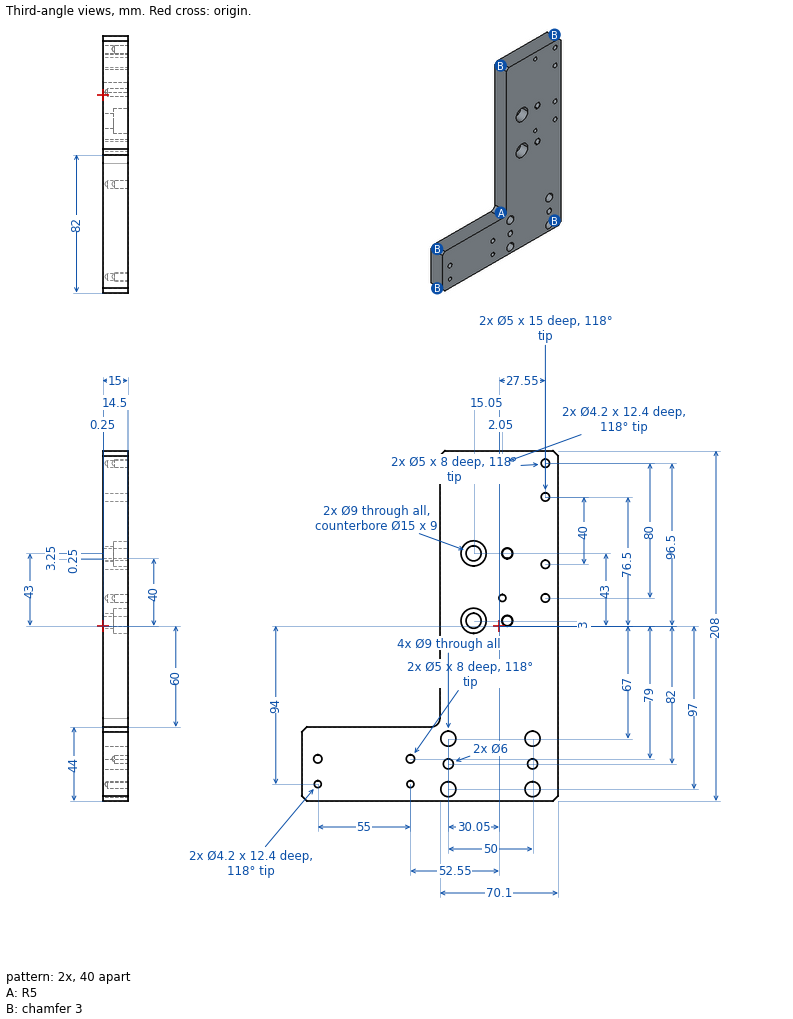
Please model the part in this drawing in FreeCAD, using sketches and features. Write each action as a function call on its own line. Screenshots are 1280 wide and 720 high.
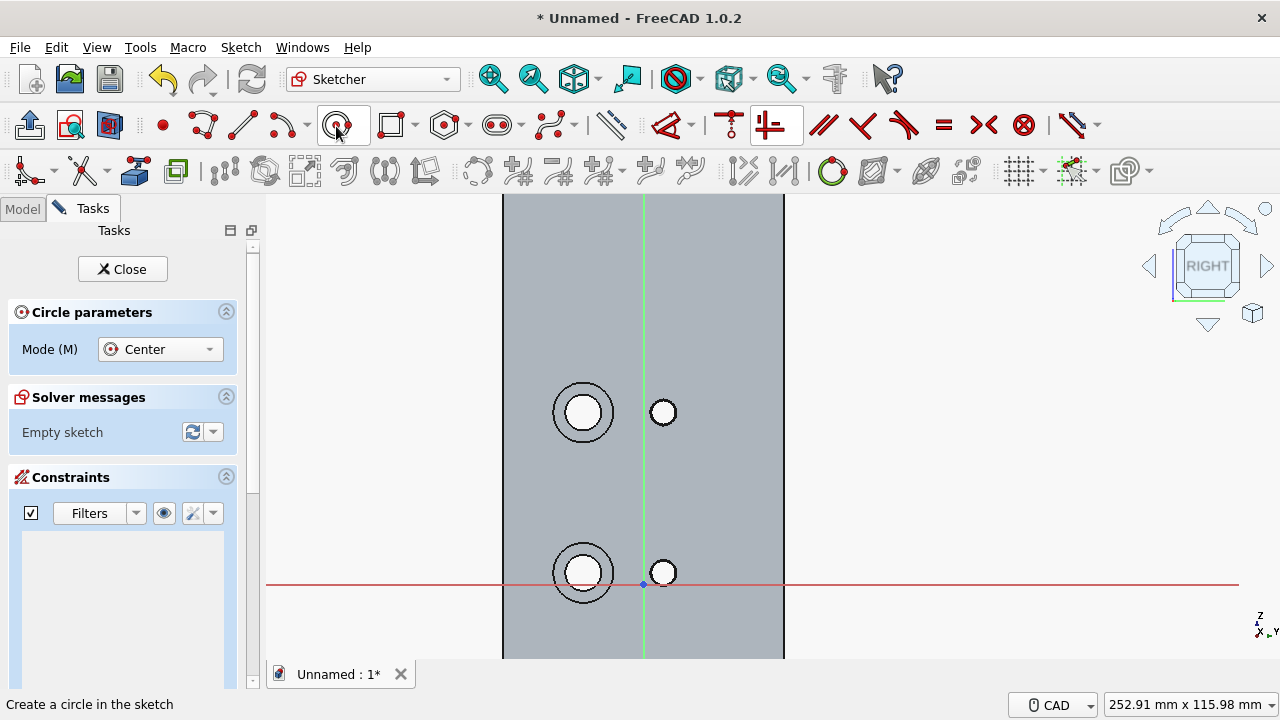
scroll(754, 278, up, 5)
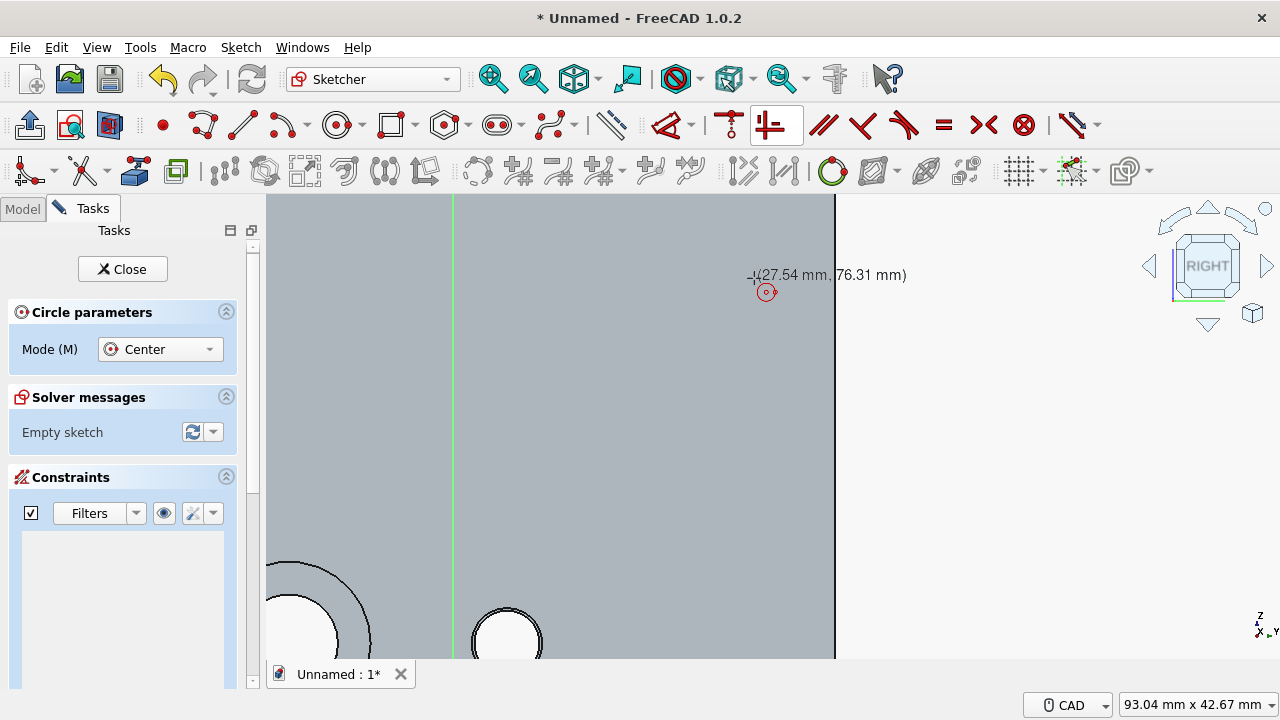
click(753, 278)
click(773, 259)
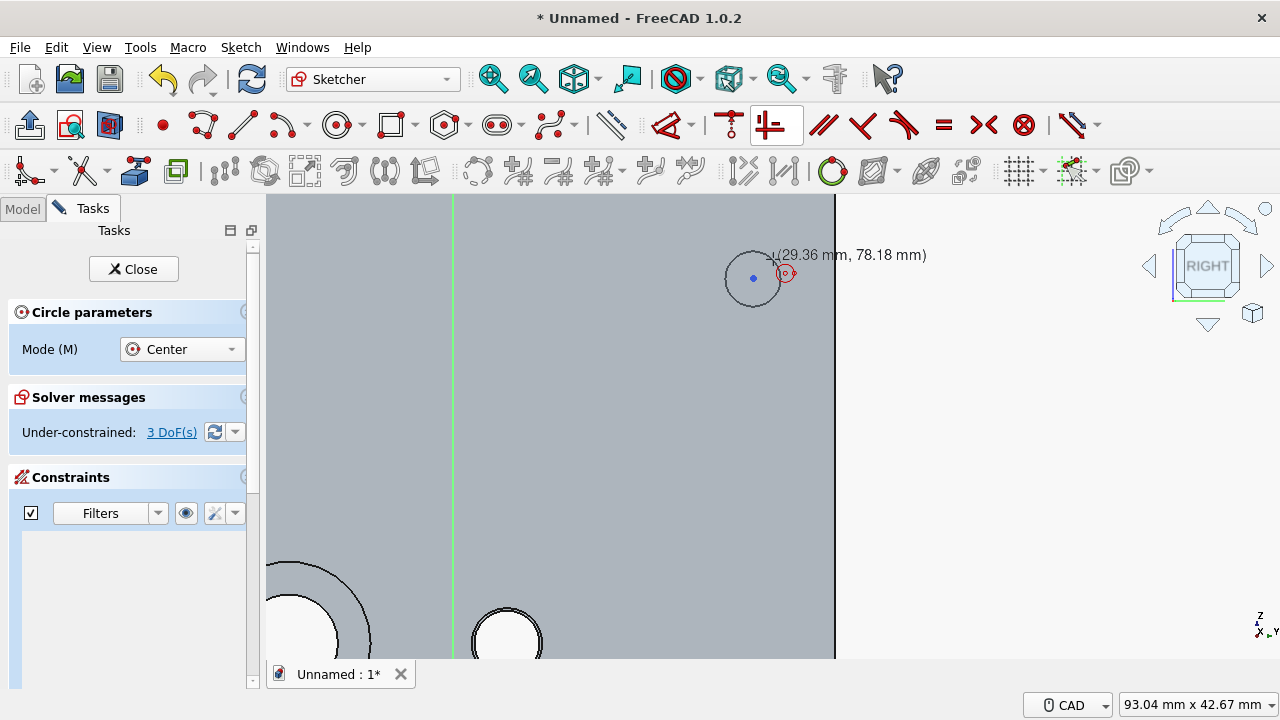
scroll(756, 278, down, 5)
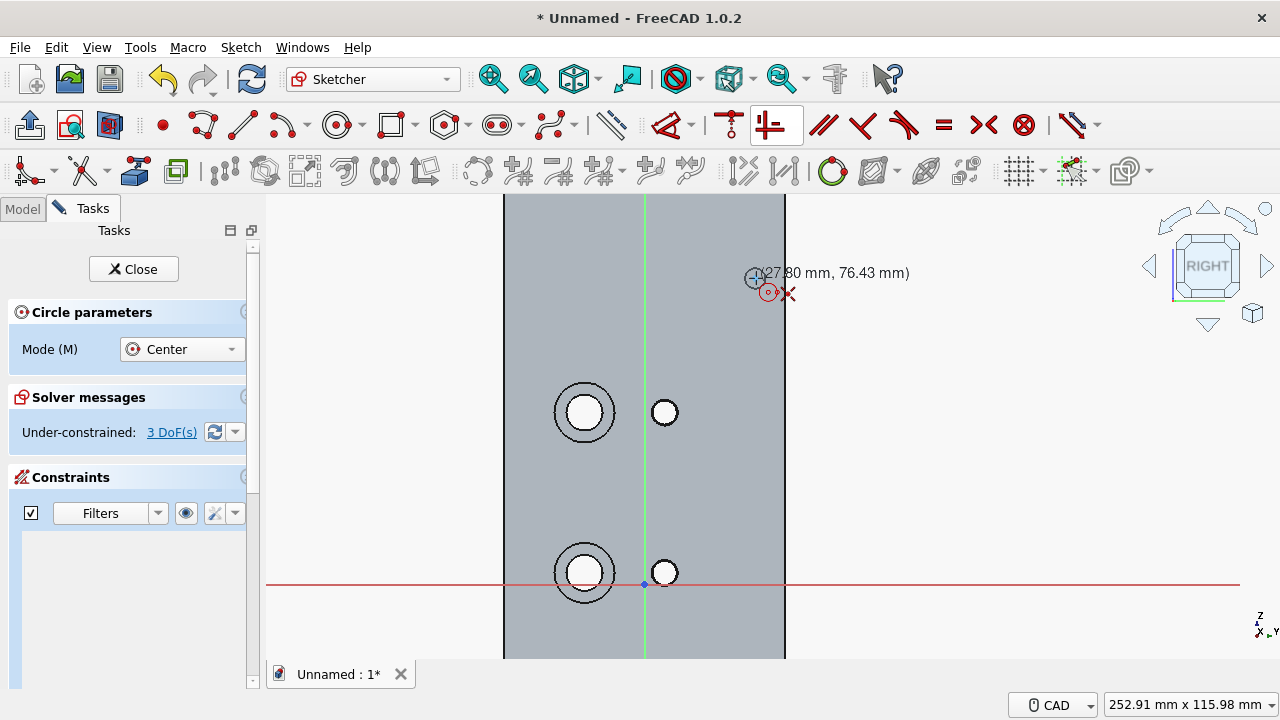
scroll(755, 439, up, 5)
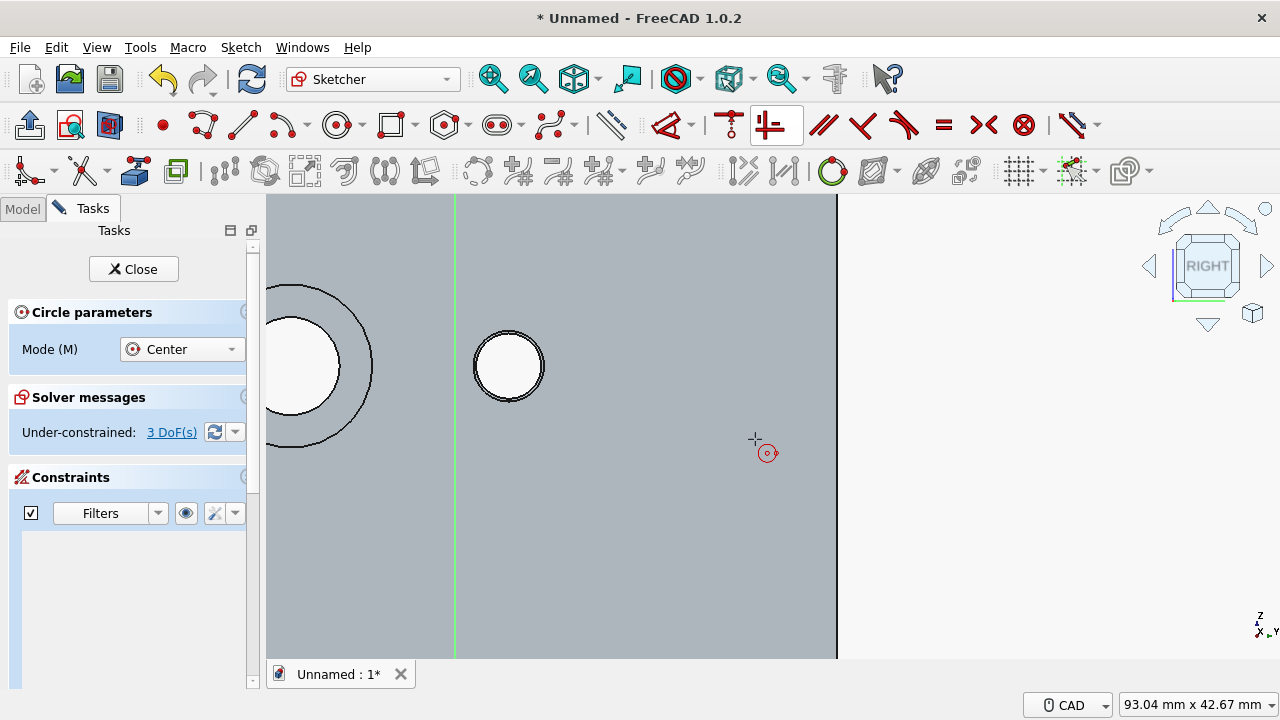
click(755, 437)
click(774, 418)
key(Escape)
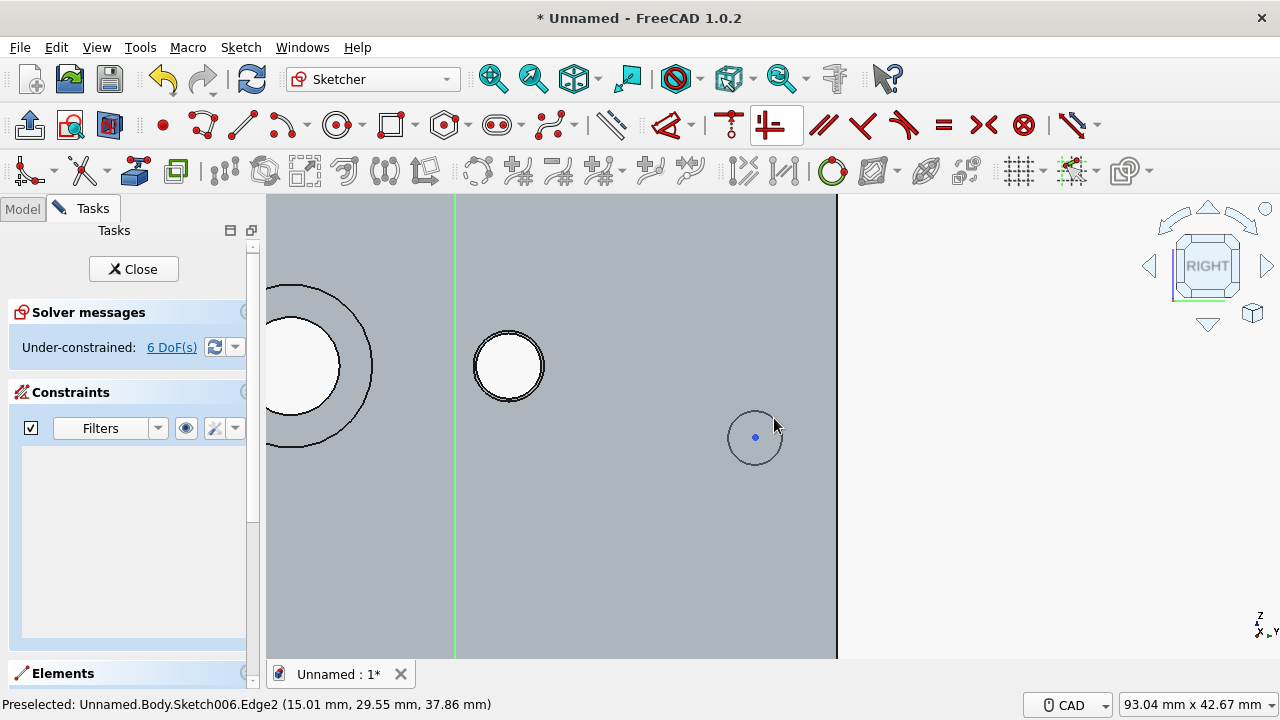
scroll(755, 439, down, 5)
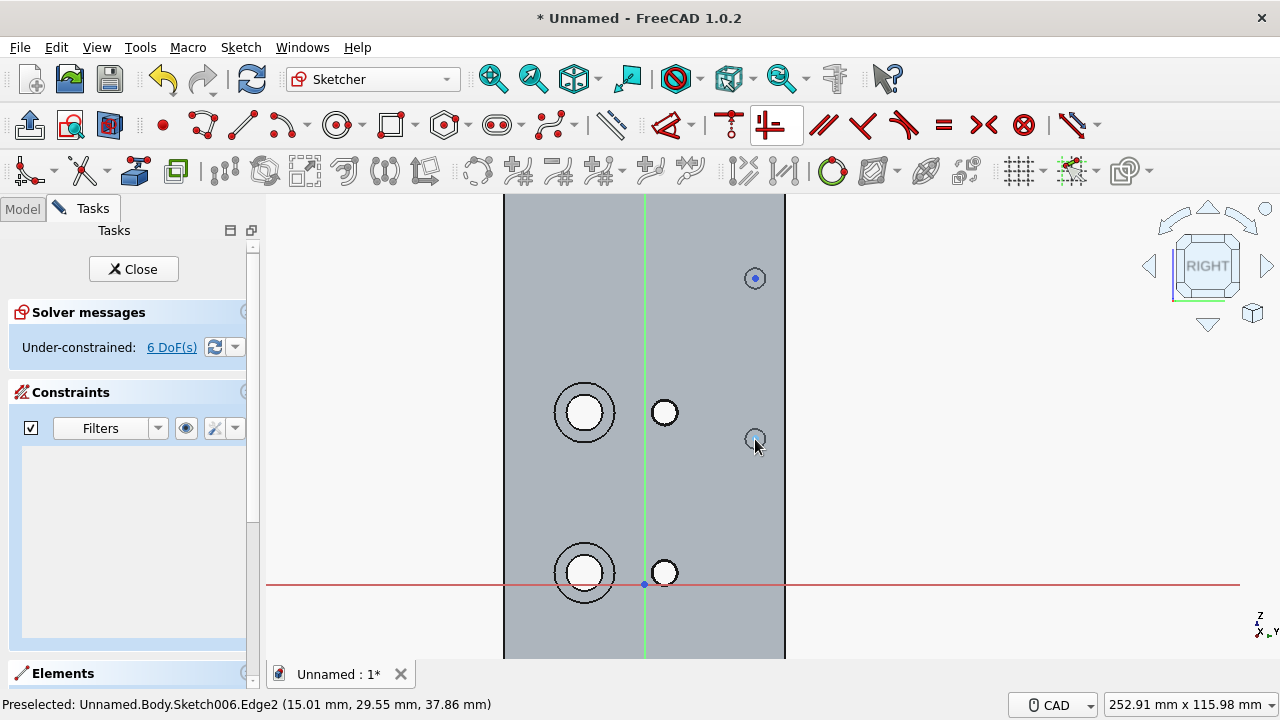
scroll(762, 271, up, 2)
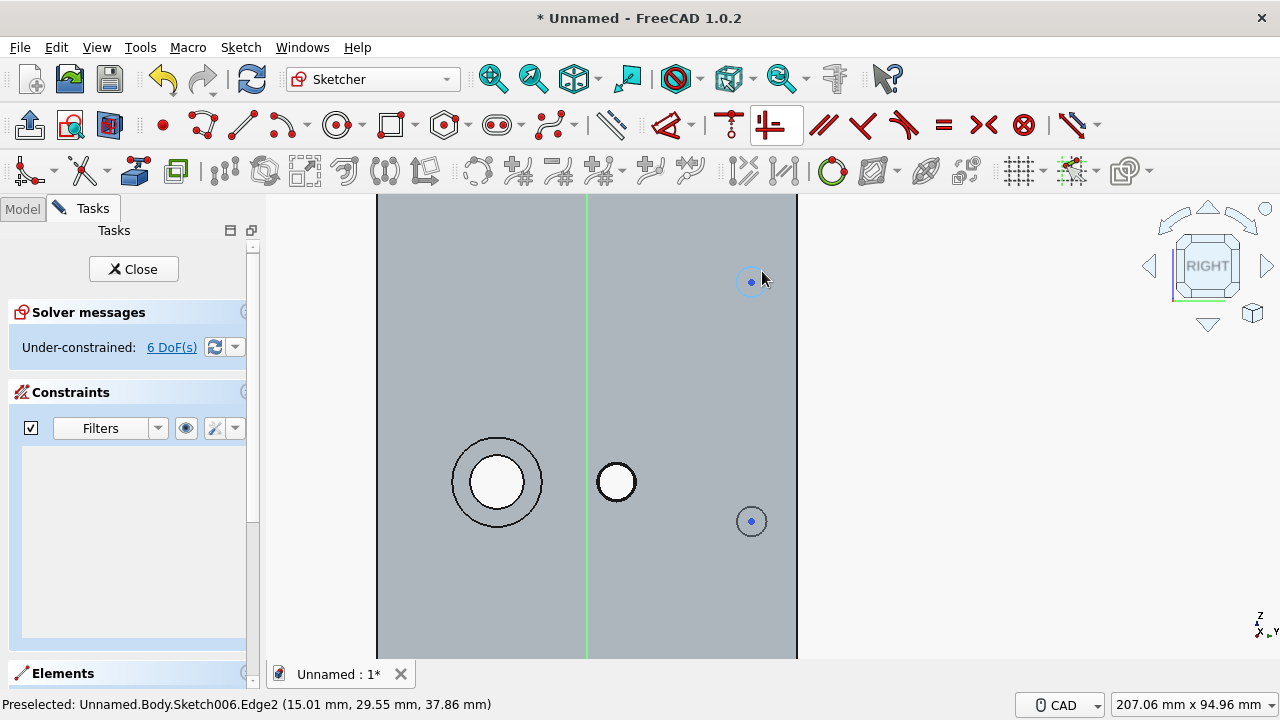
click(762, 271)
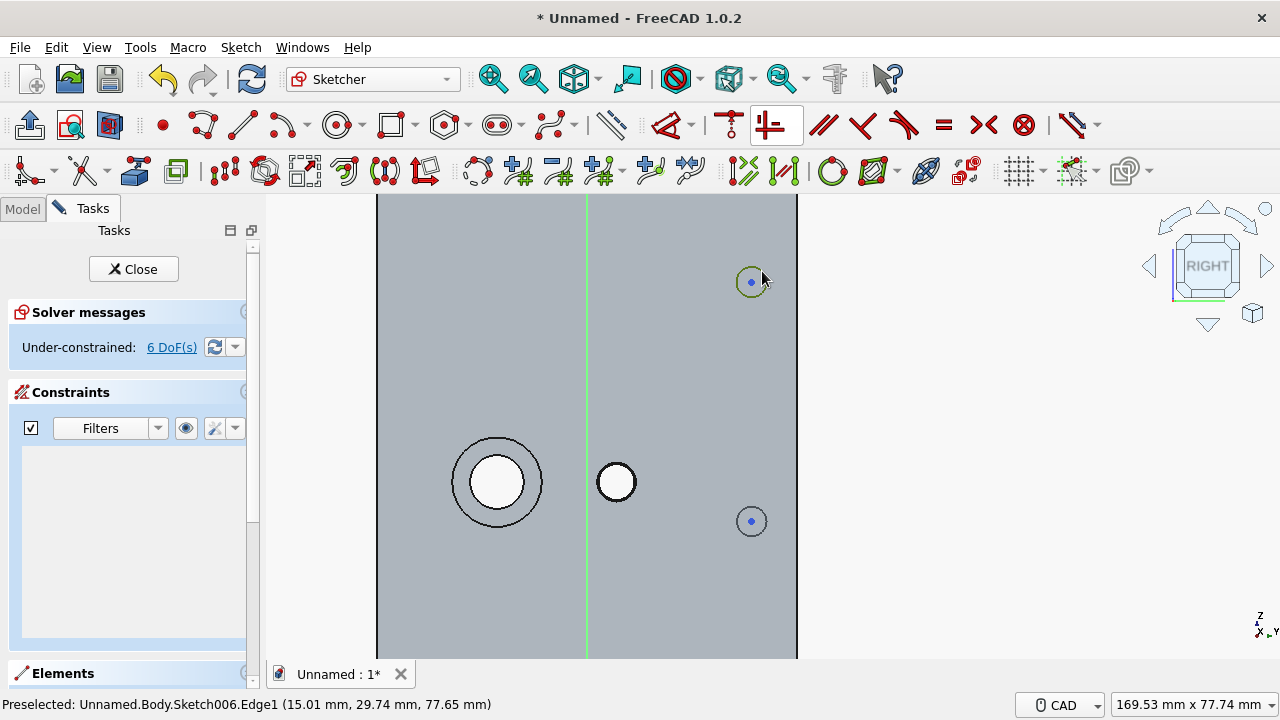
click(762, 511)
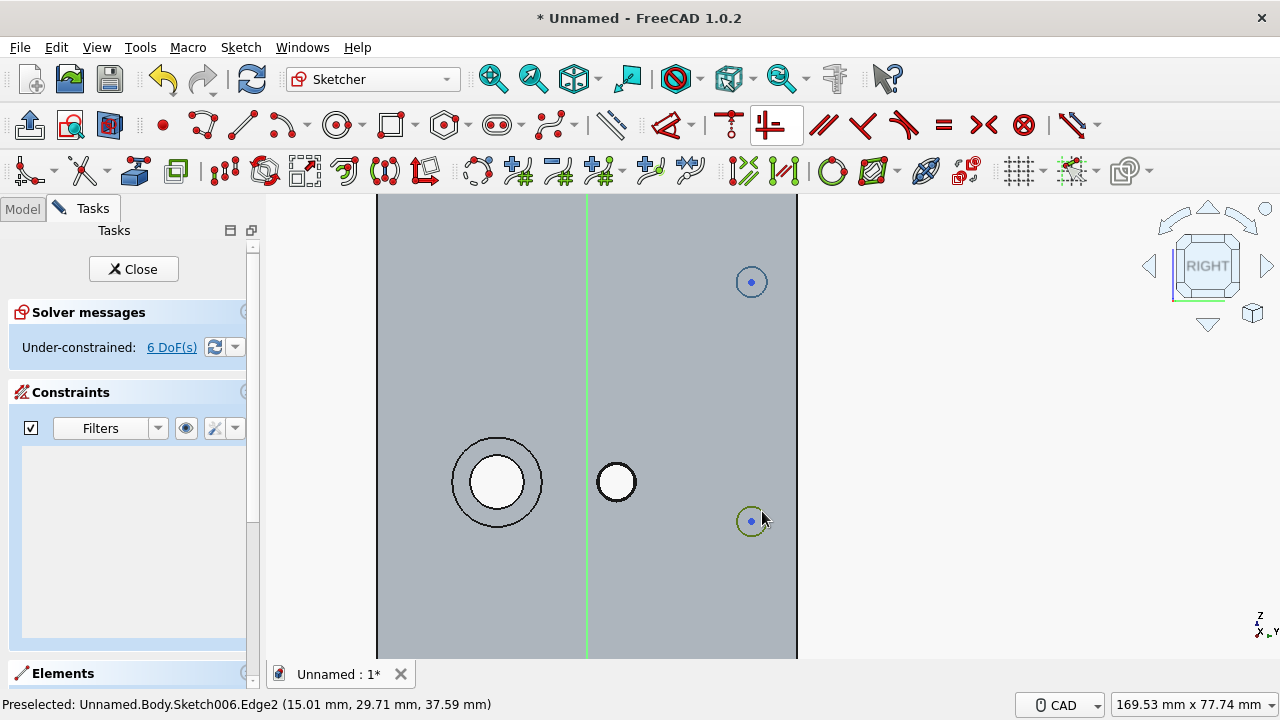
click(944, 126)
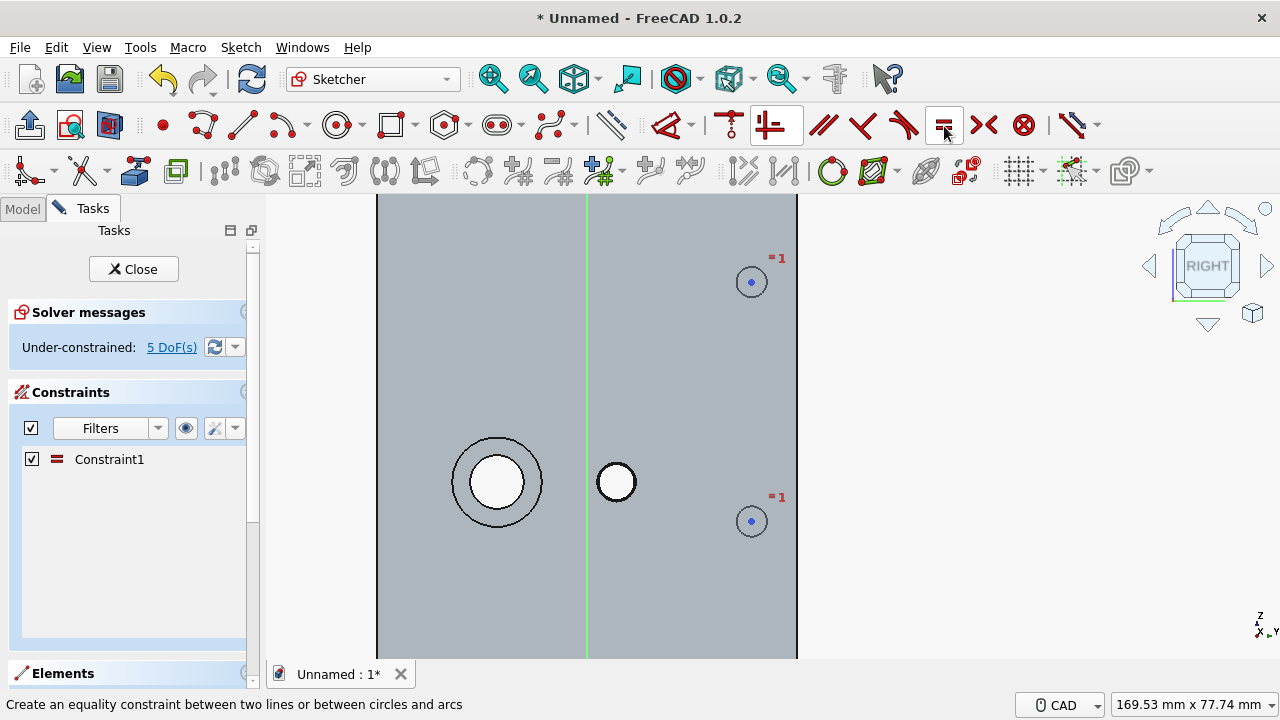
click(752, 282)